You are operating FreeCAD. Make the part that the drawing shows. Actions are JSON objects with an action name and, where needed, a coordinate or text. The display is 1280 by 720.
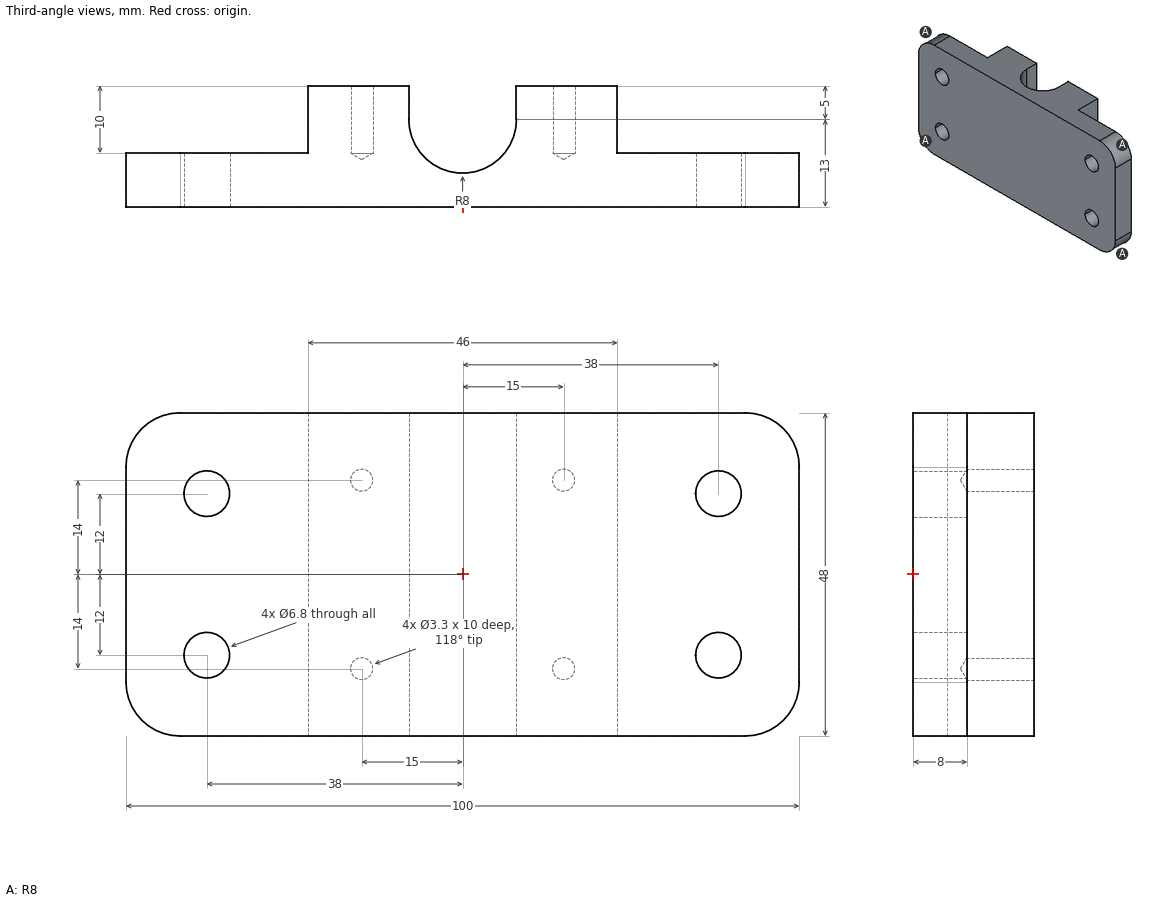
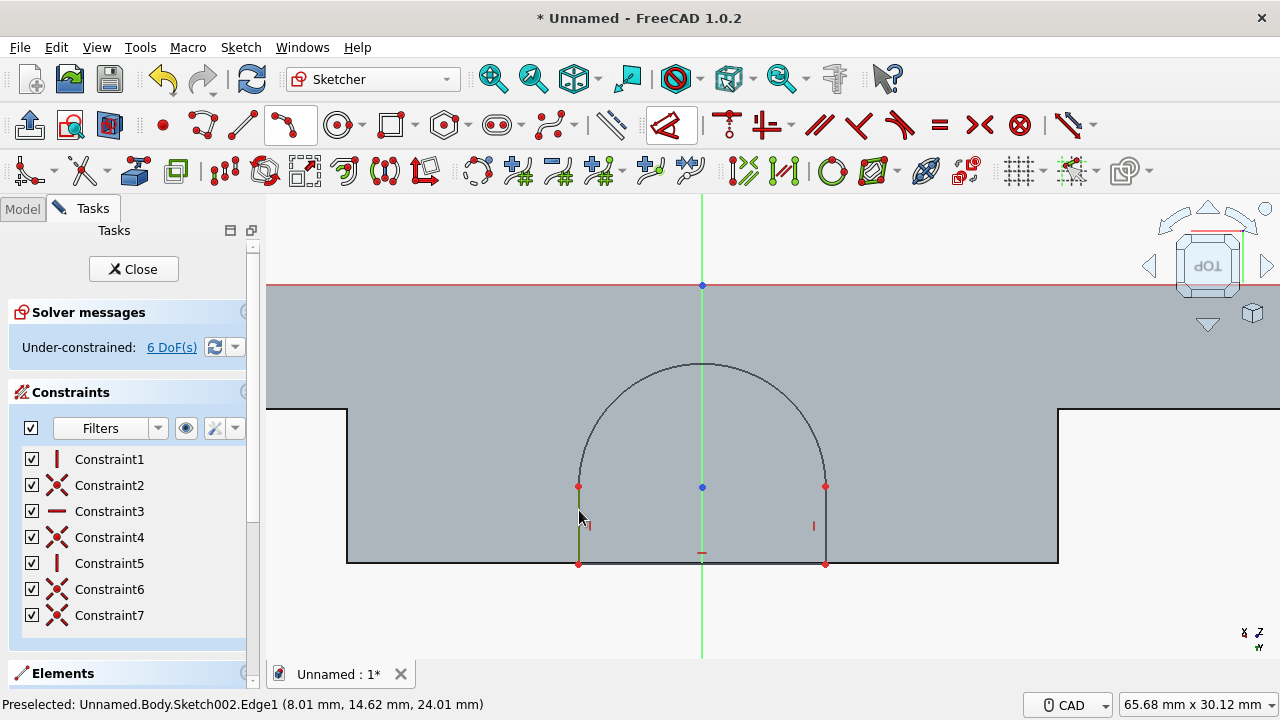
{"action": "left_click", "coordinate": [775, 387]}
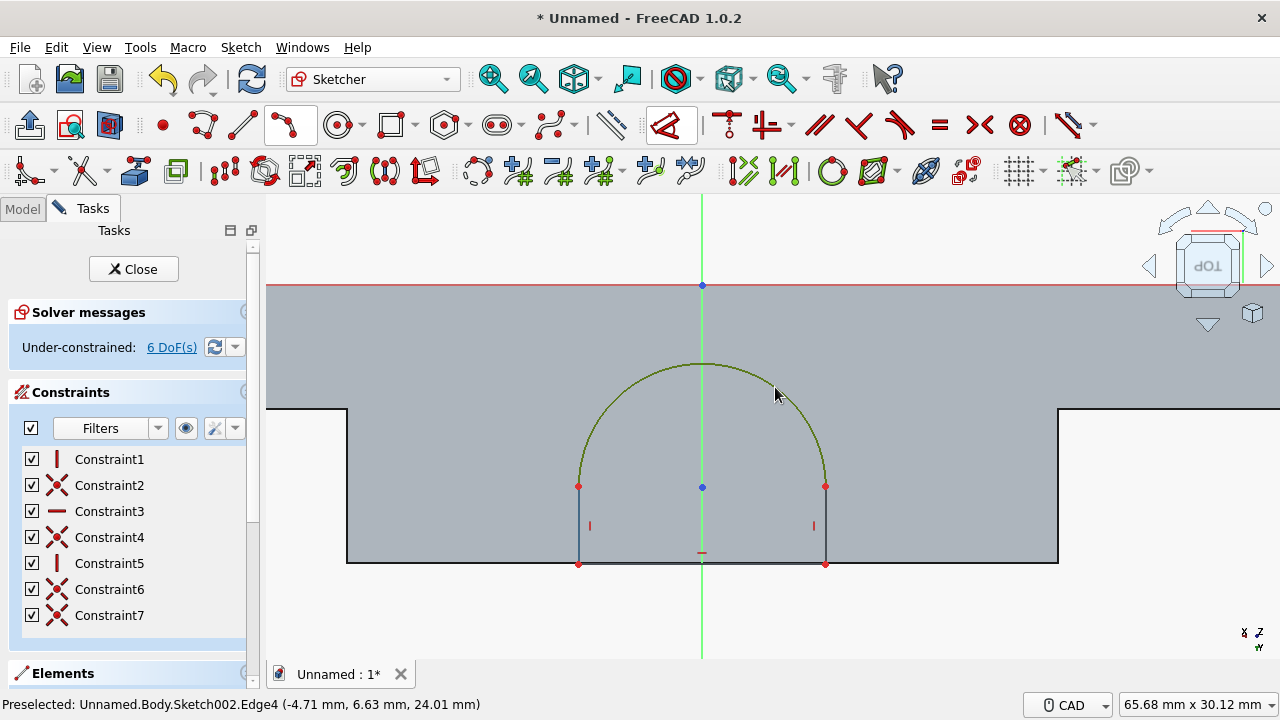
{"action": "left_click", "coordinate": [900, 126]}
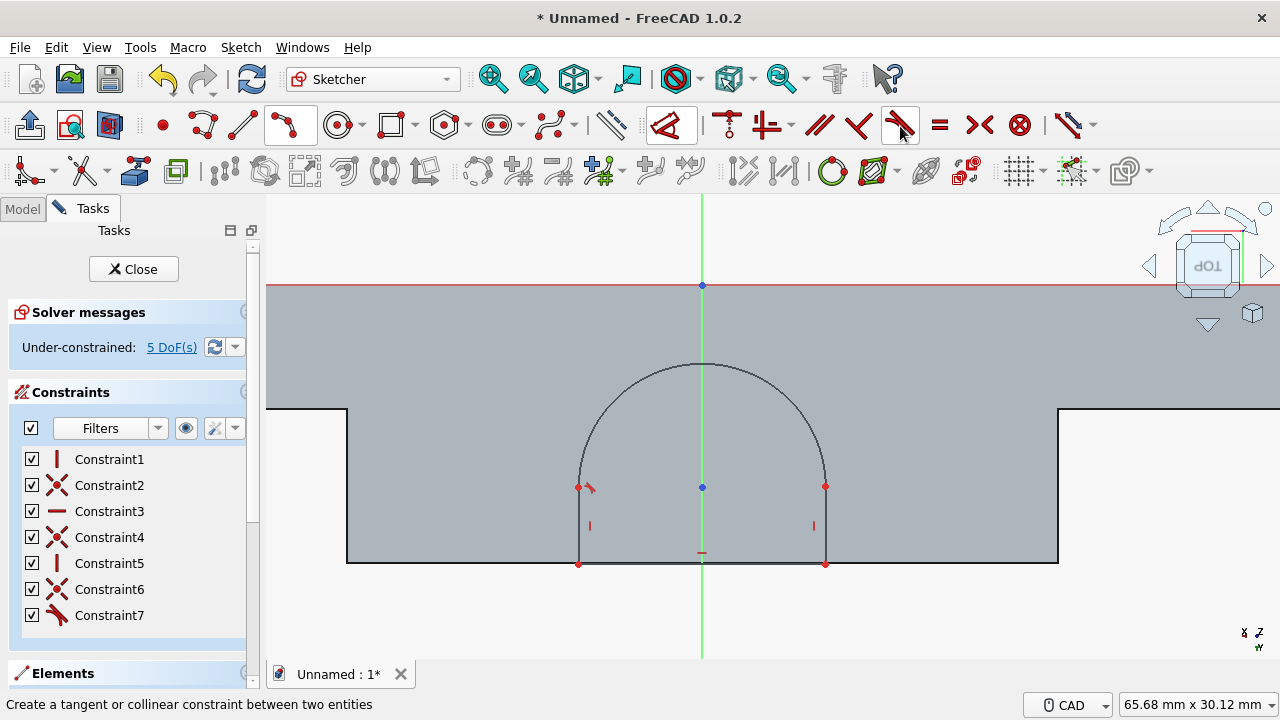
{"action": "left_click", "coordinate": [826, 541]}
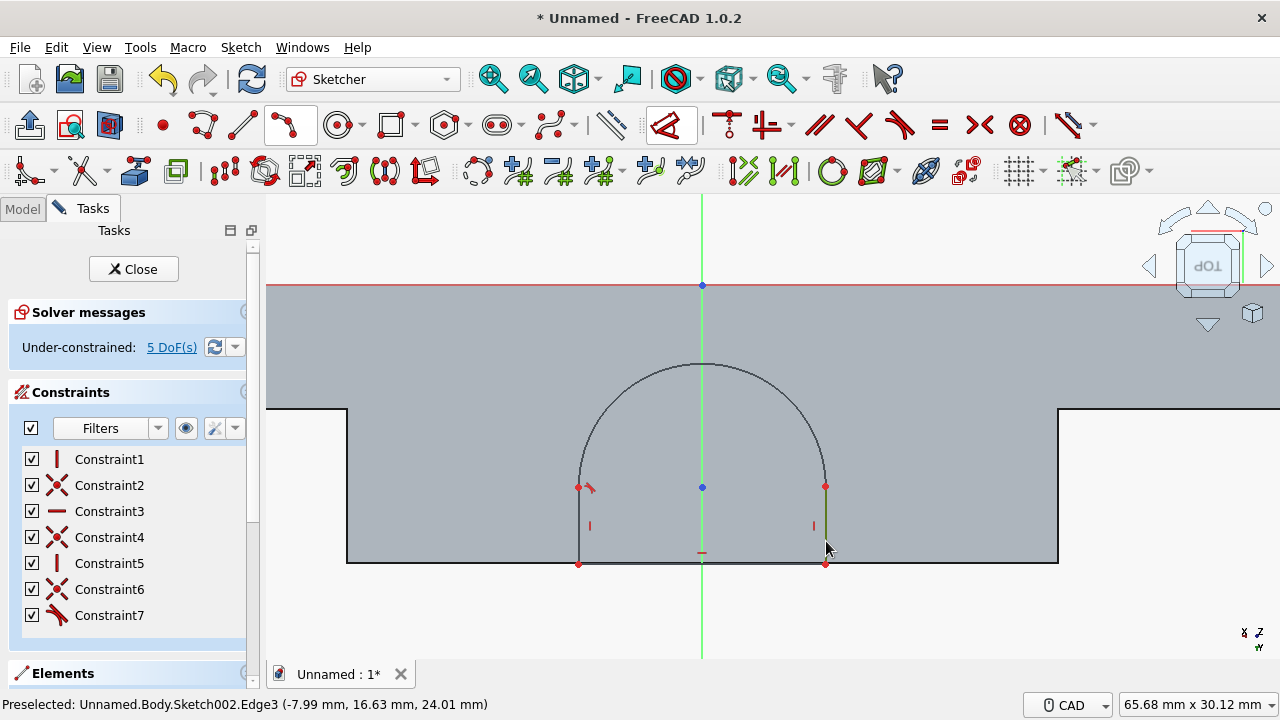
{"action": "left_click", "coordinate": [775, 387]}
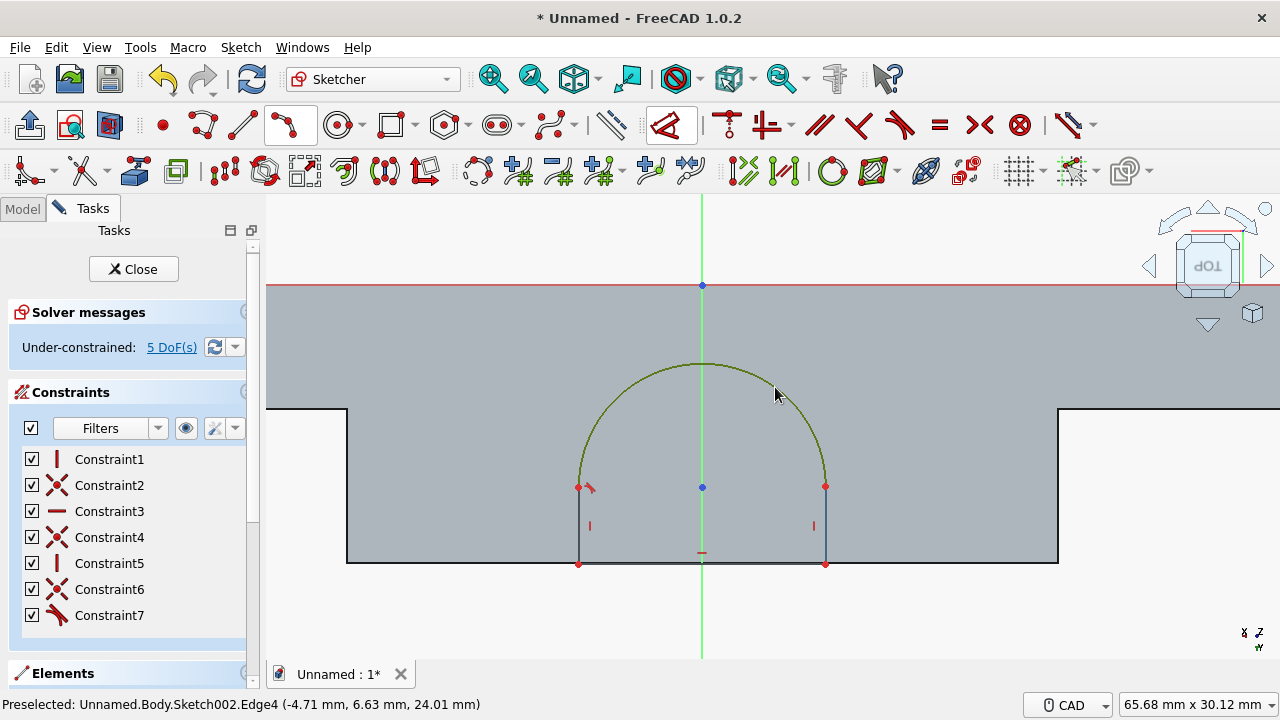
{"action": "key", "text": "t"}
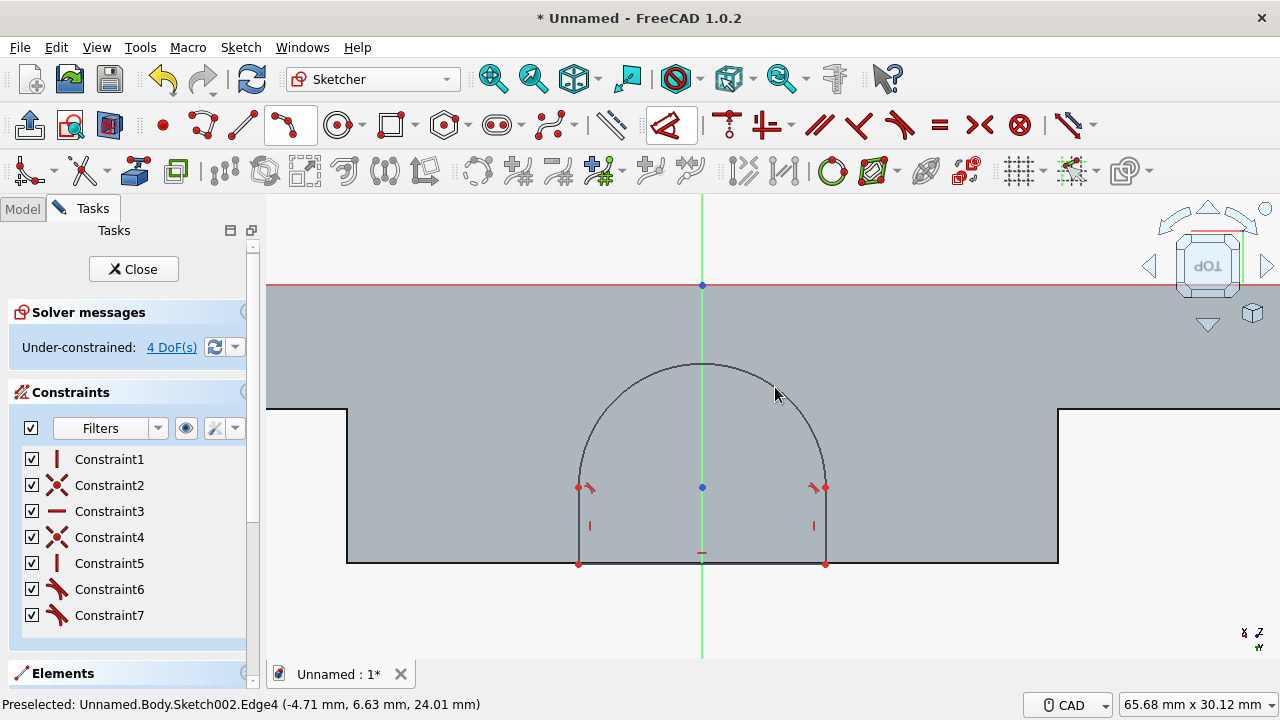
{"action": "left_click", "coordinate": [702, 487]}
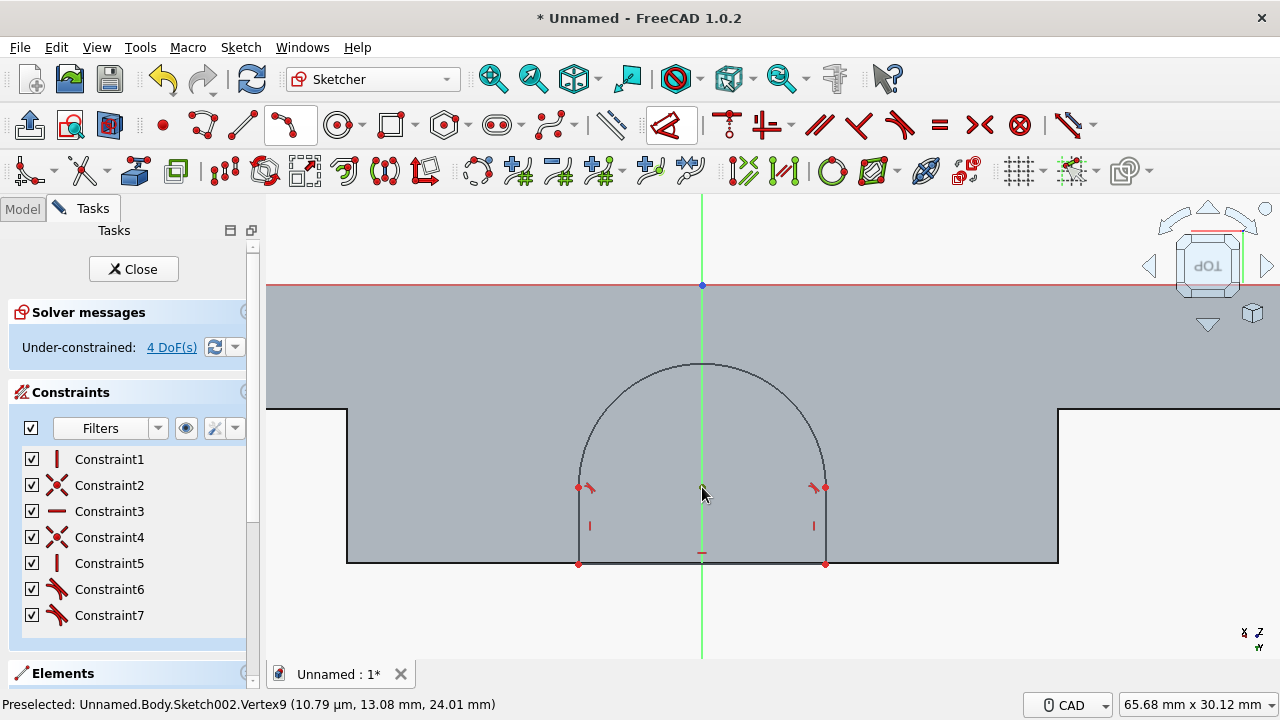
{"action": "left_click", "coordinate": [702, 602]}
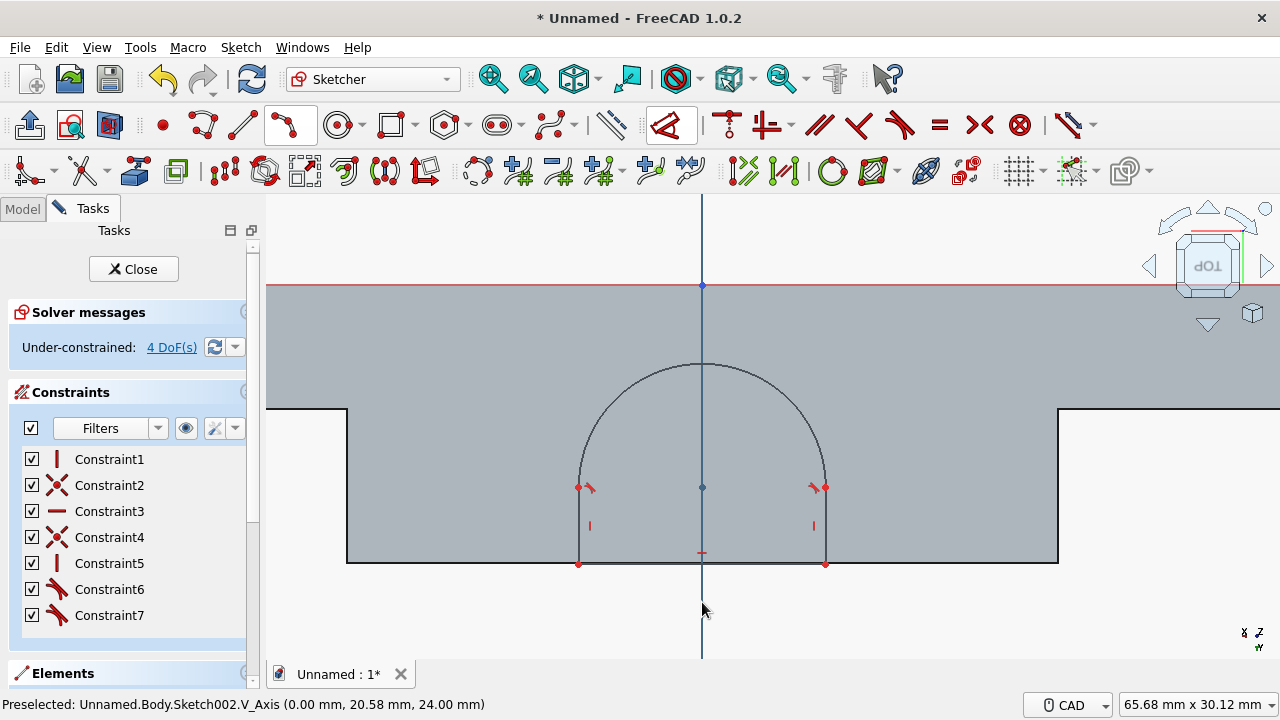
{"action": "left_click", "coordinate": [728, 126]}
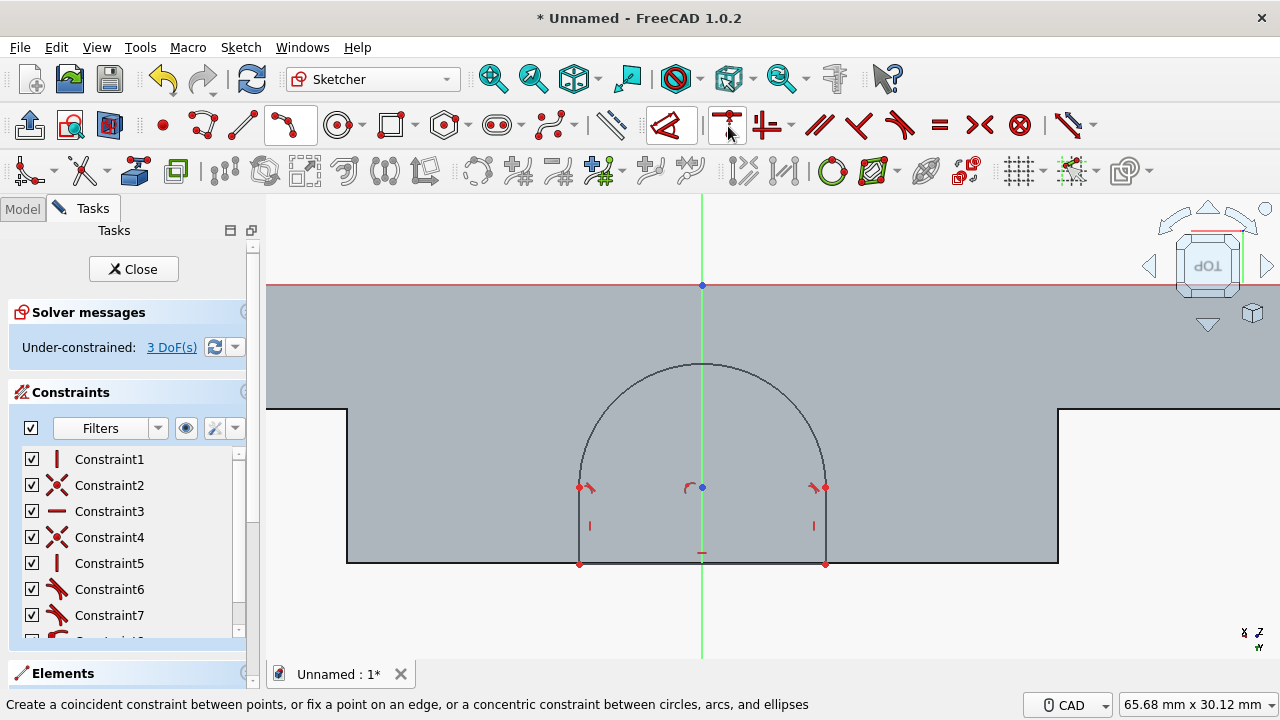
{"action": "left_click", "coordinate": [775, 387]}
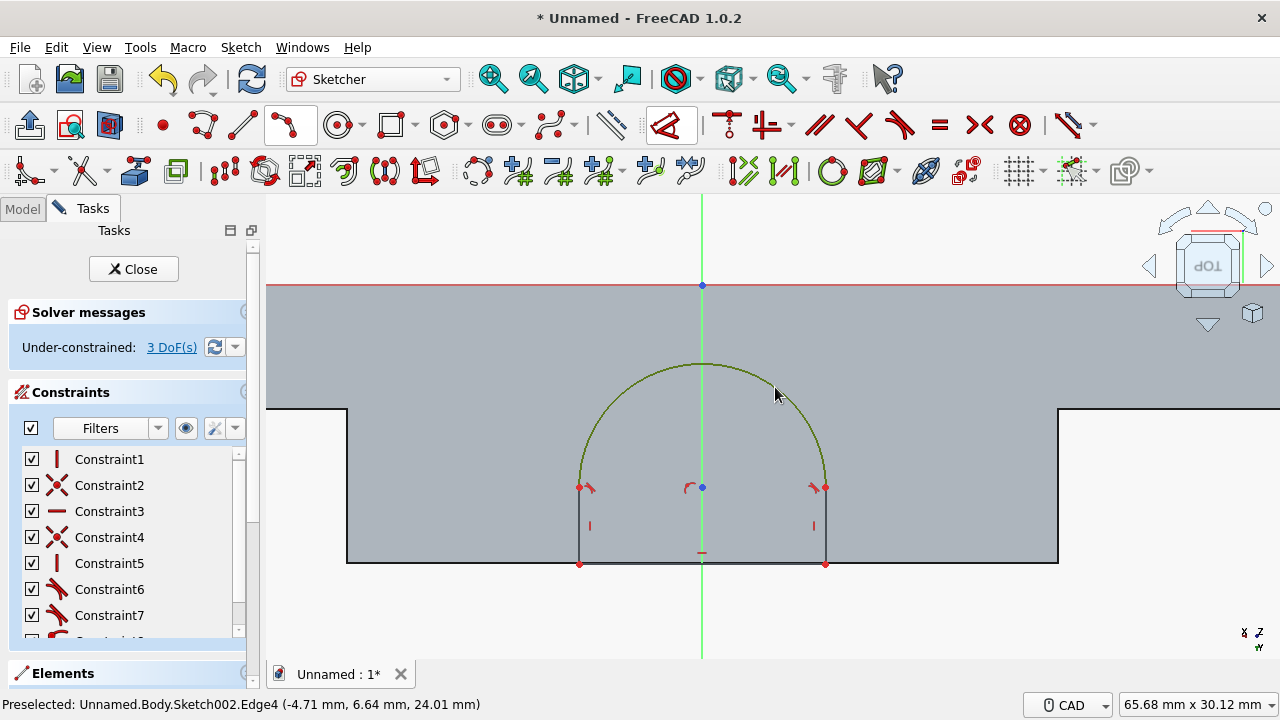
{"action": "key", "text": "k r"}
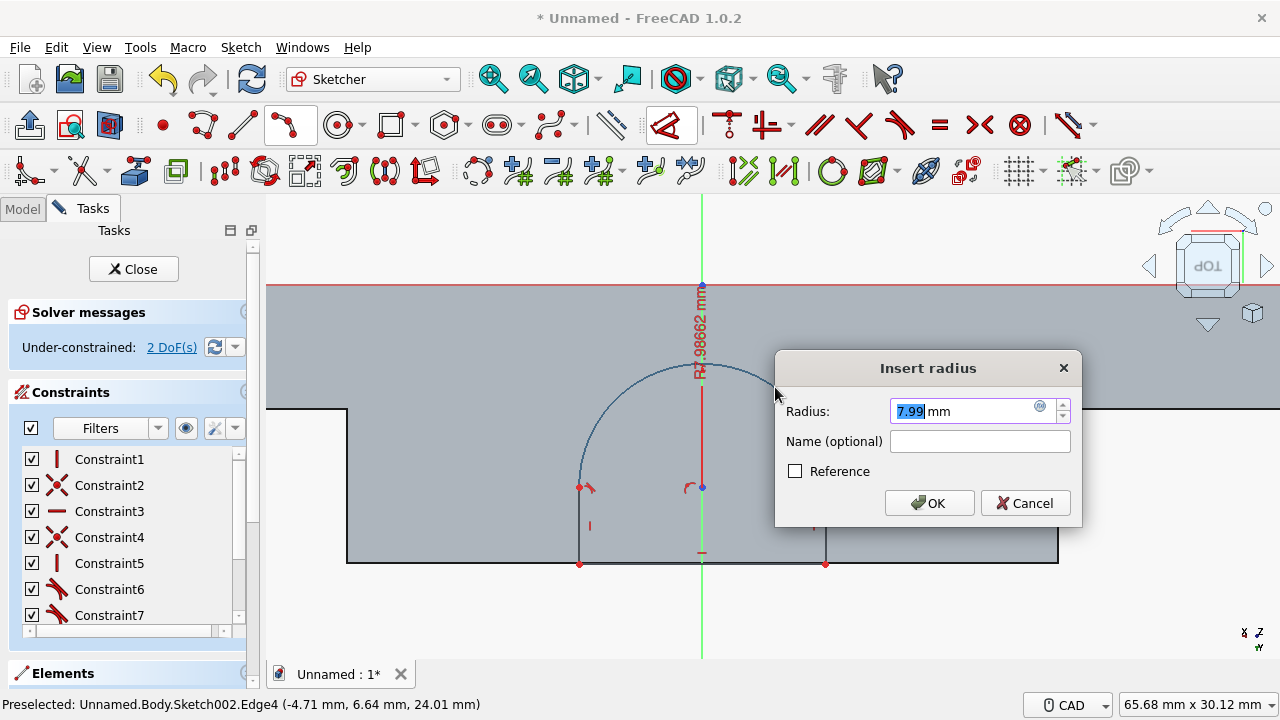
{"action": "type", "text": "8"}
{"action": "key", "text": "Return"}